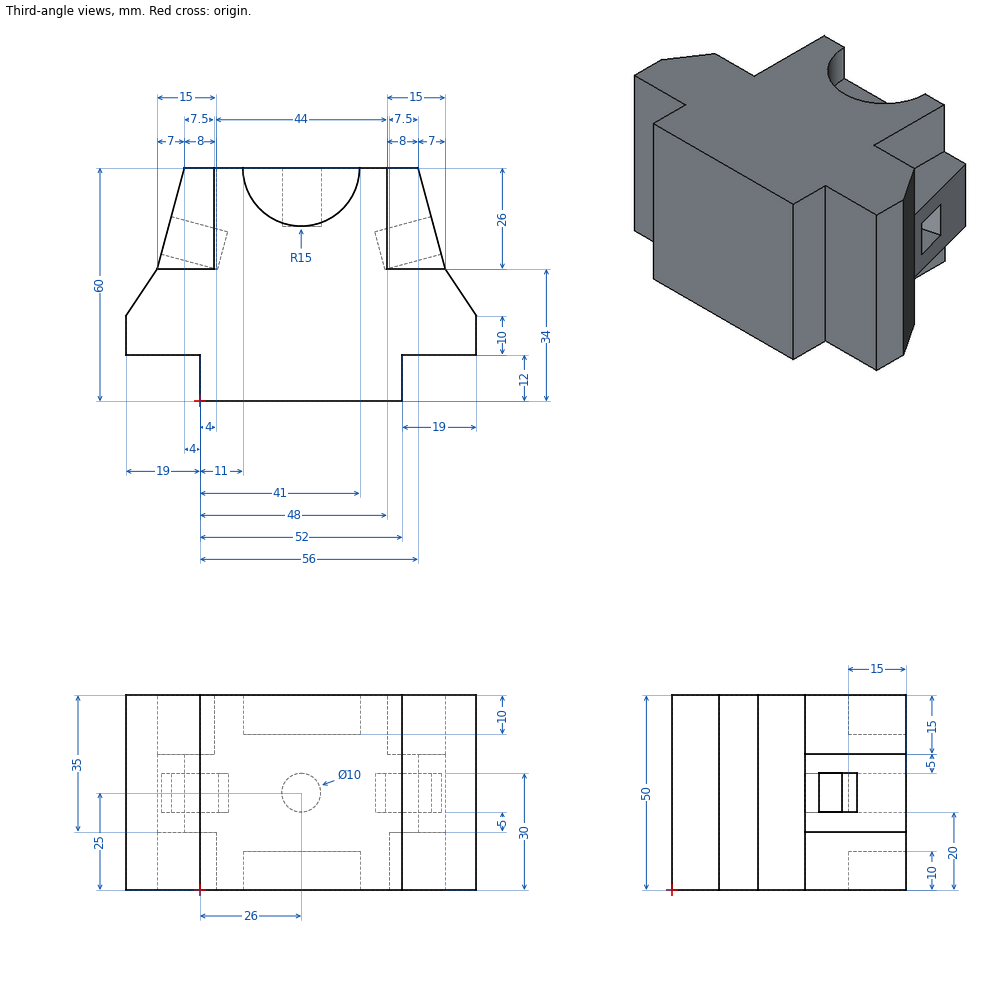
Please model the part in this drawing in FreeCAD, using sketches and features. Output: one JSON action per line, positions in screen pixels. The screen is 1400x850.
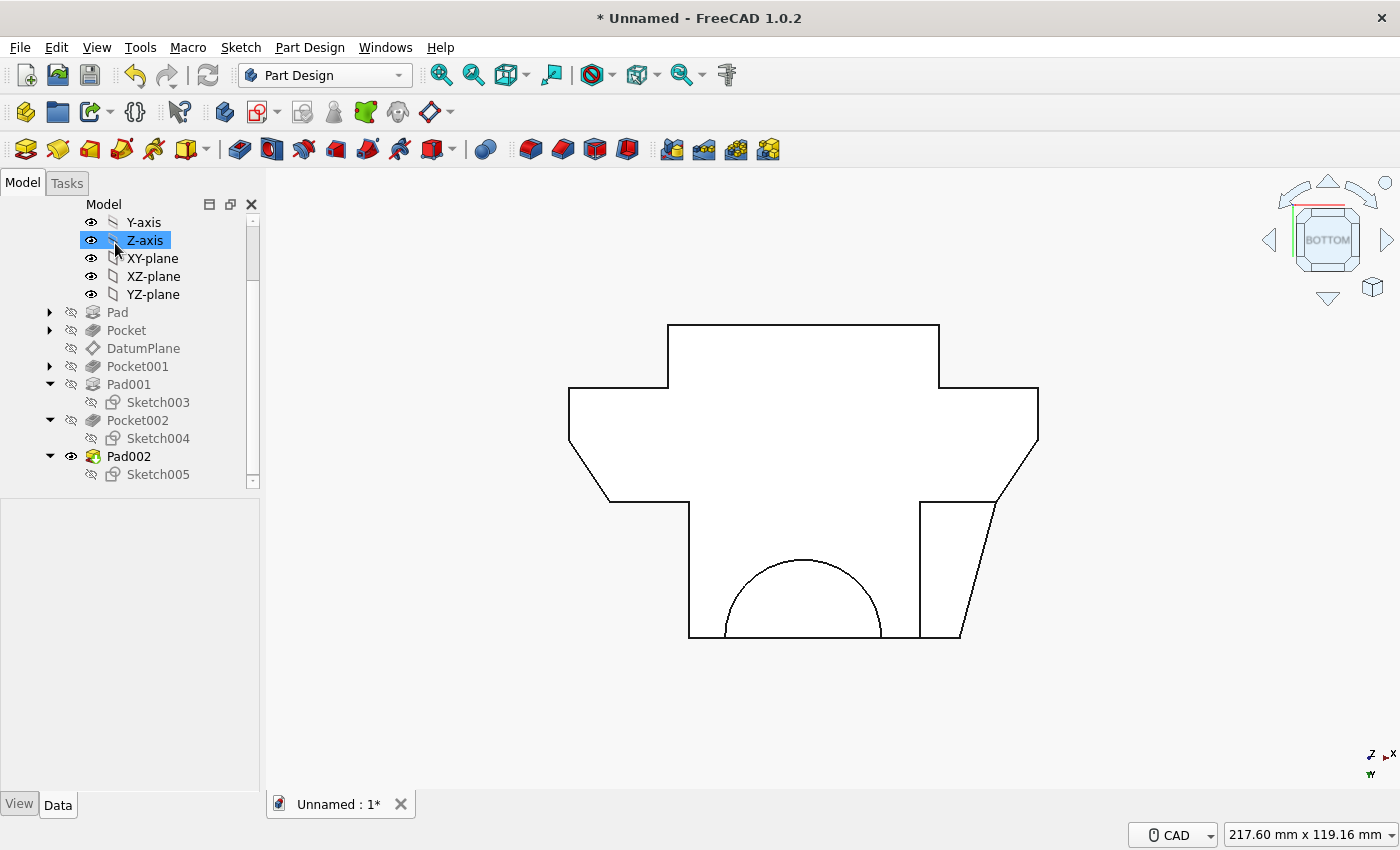
{"action": "key", "text": "0"}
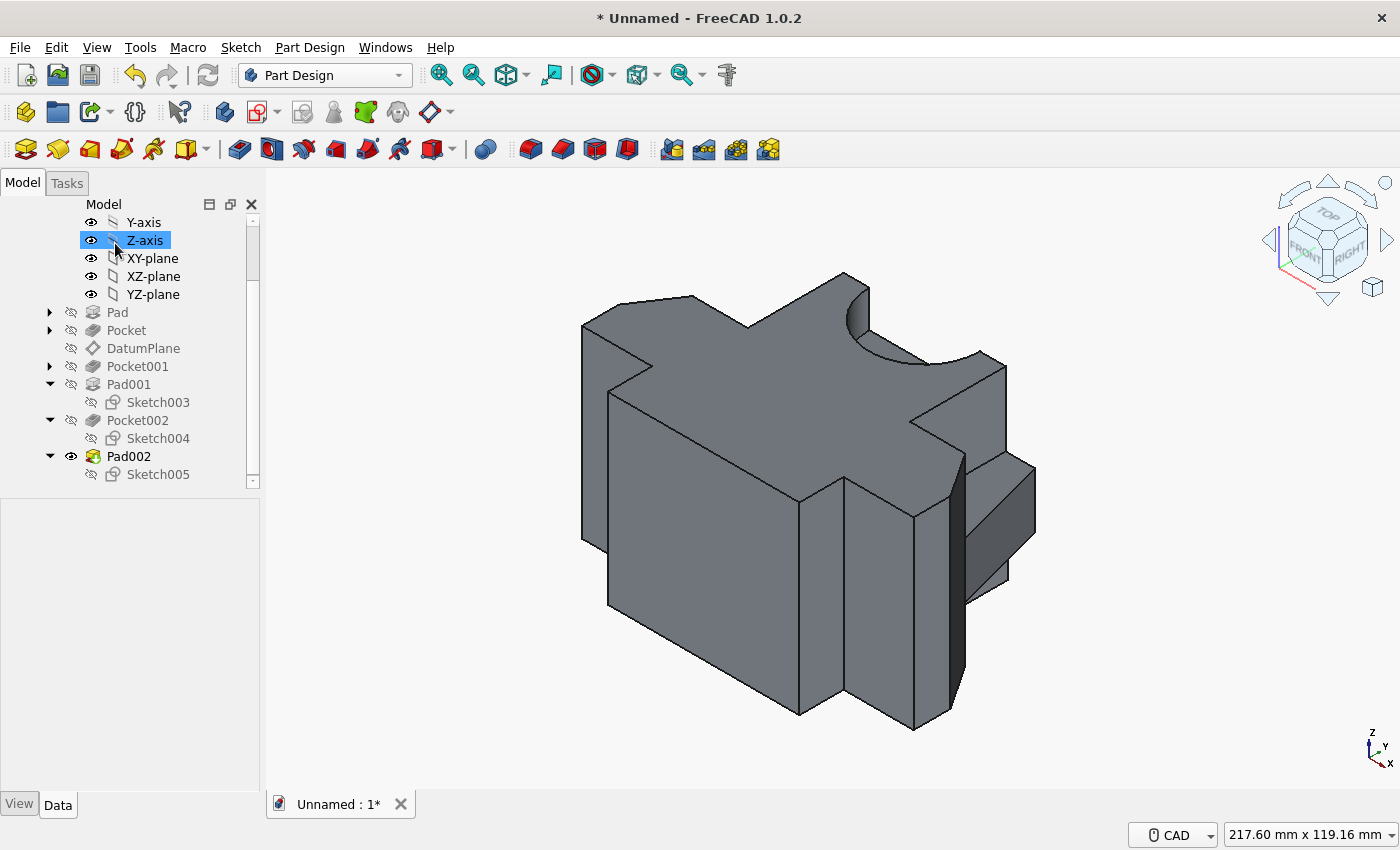
{"action": "left_click", "coordinate": [978, 490]}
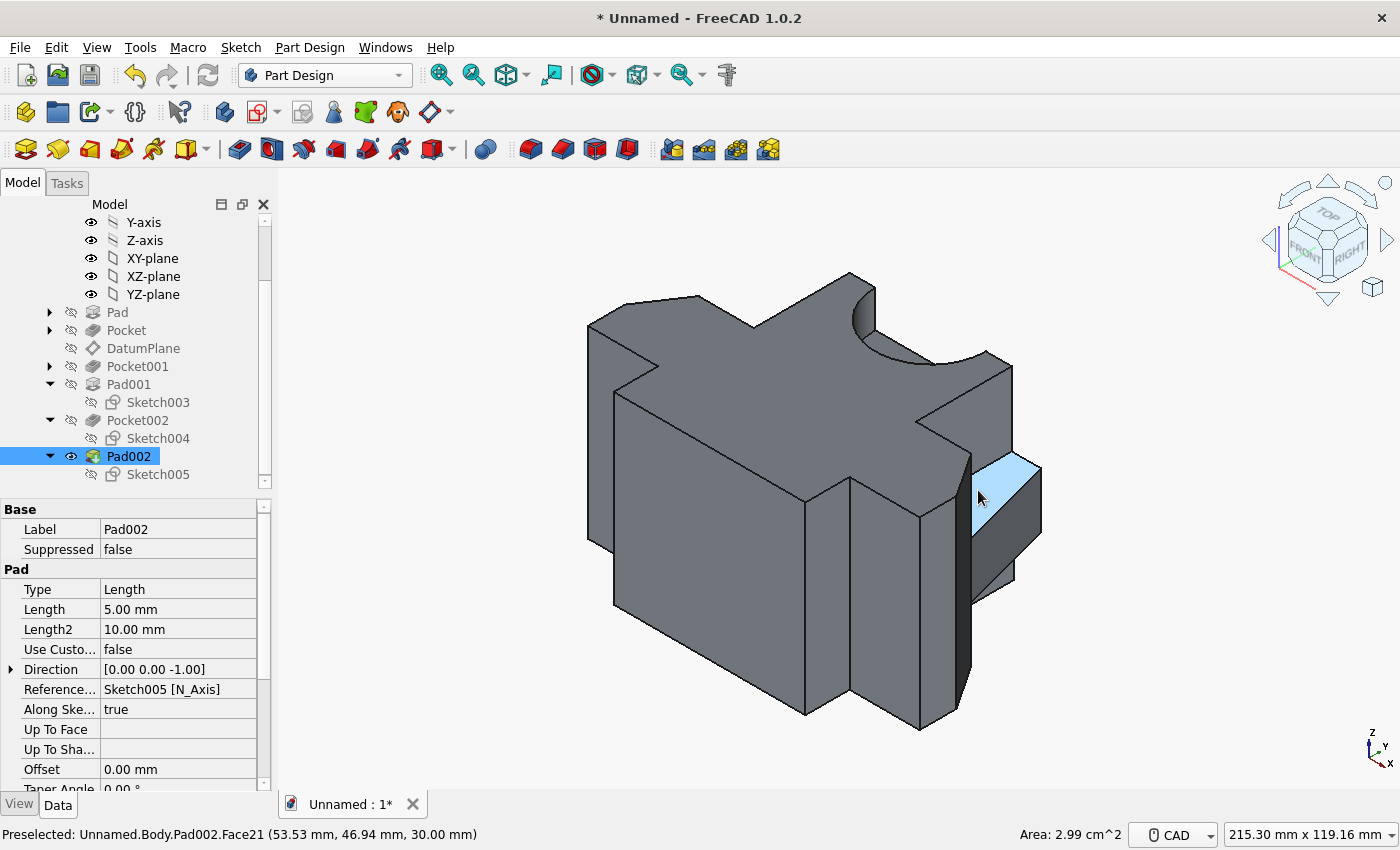
{"action": "left_click", "coordinate": [258, 112]}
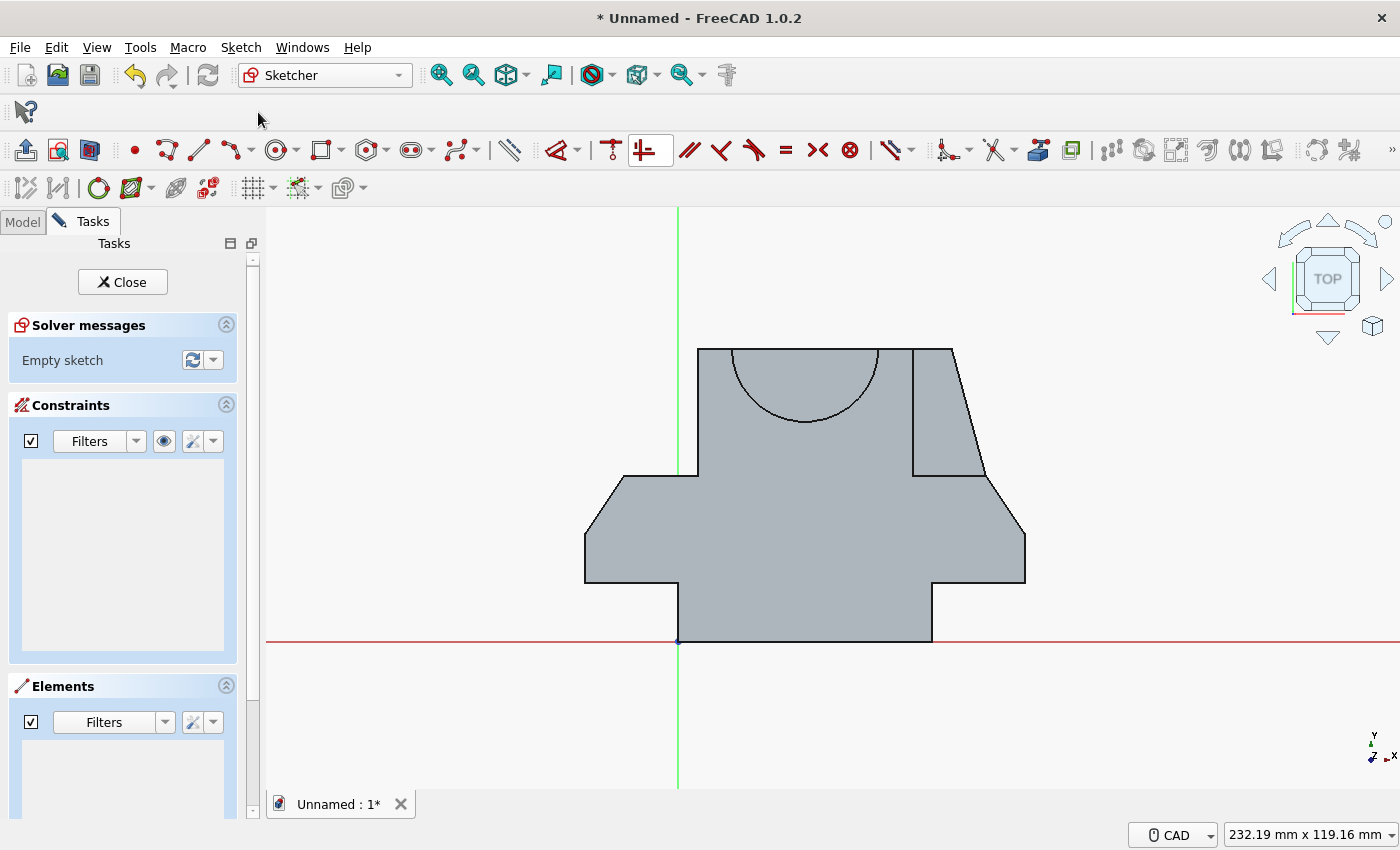
{"action": "left_click", "coordinate": [90, 150]}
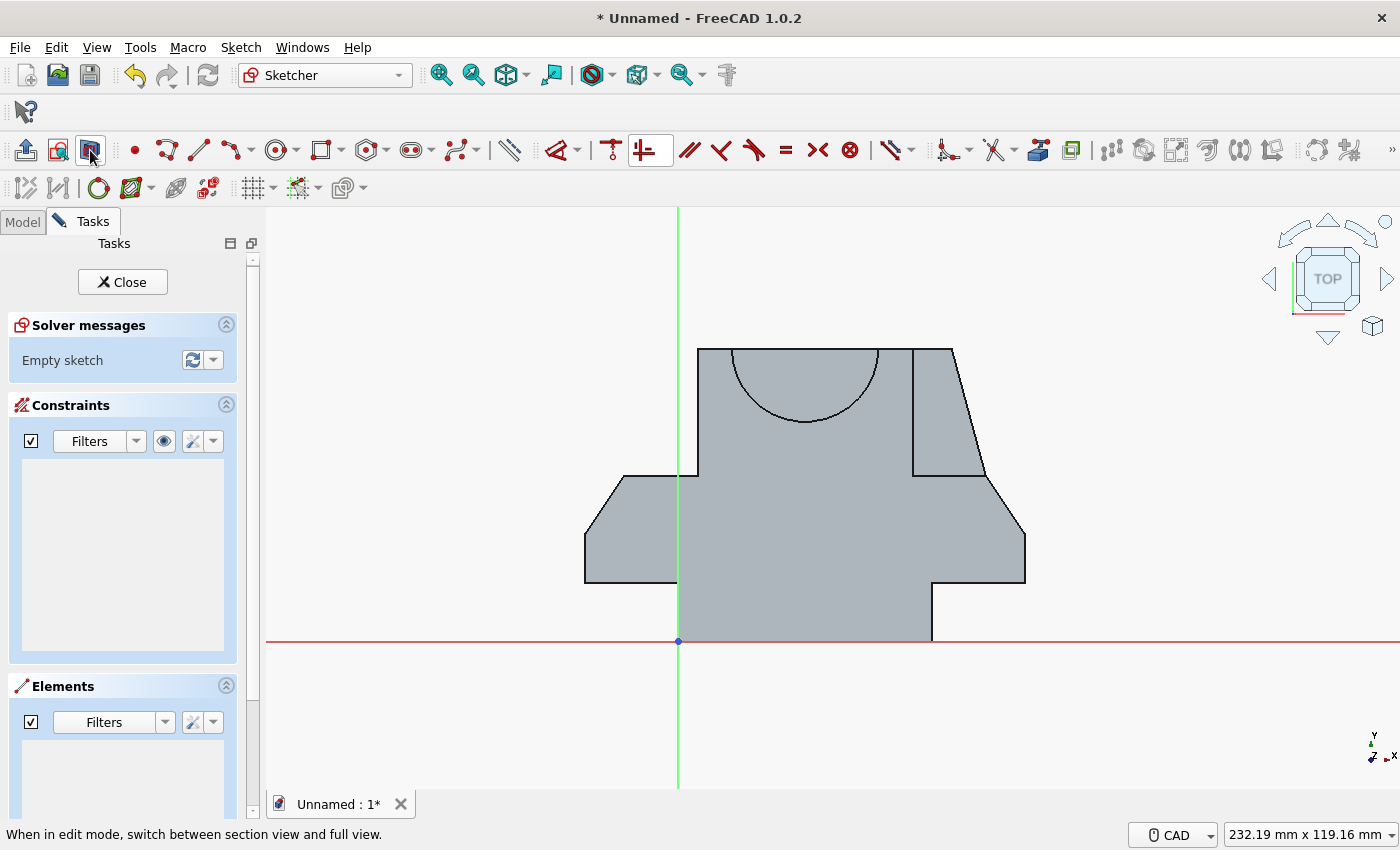
{"action": "left_click", "coordinate": [168, 150]}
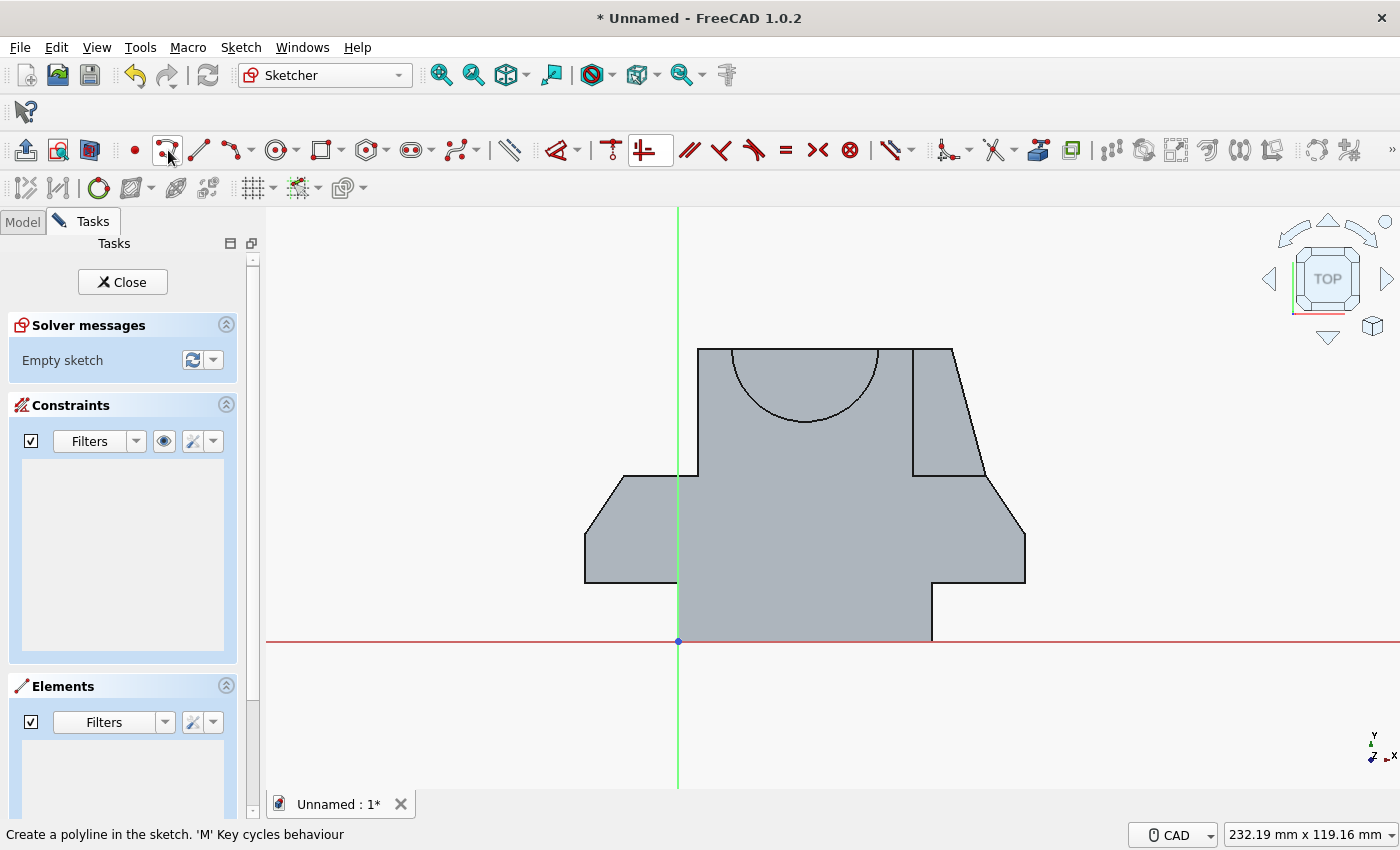
{"action": "left_click", "coordinate": [913, 476]}
{"action": "left_click", "coordinate": [986, 476]}
{"action": "left_click", "coordinate": [952, 349]}
{"action": "left_click", "coordinate": [913, 349]}
{"action": "left_click", "coordinate": [913, 477]}
{"action": "key", "text": "Escape"}
{"action": "key", "text": "Escape"}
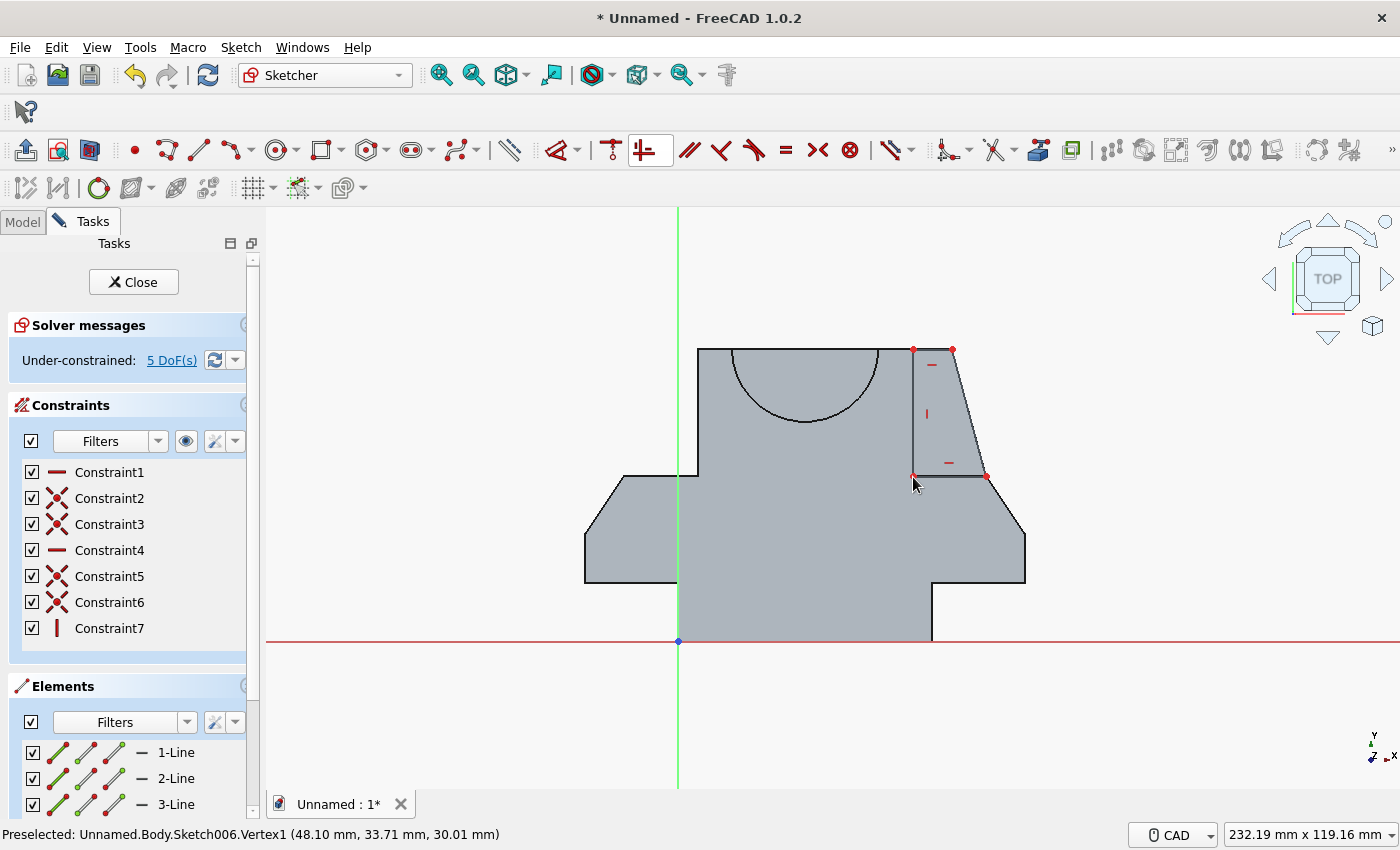
{"action": "left_click", "coordinate": [556, 150]}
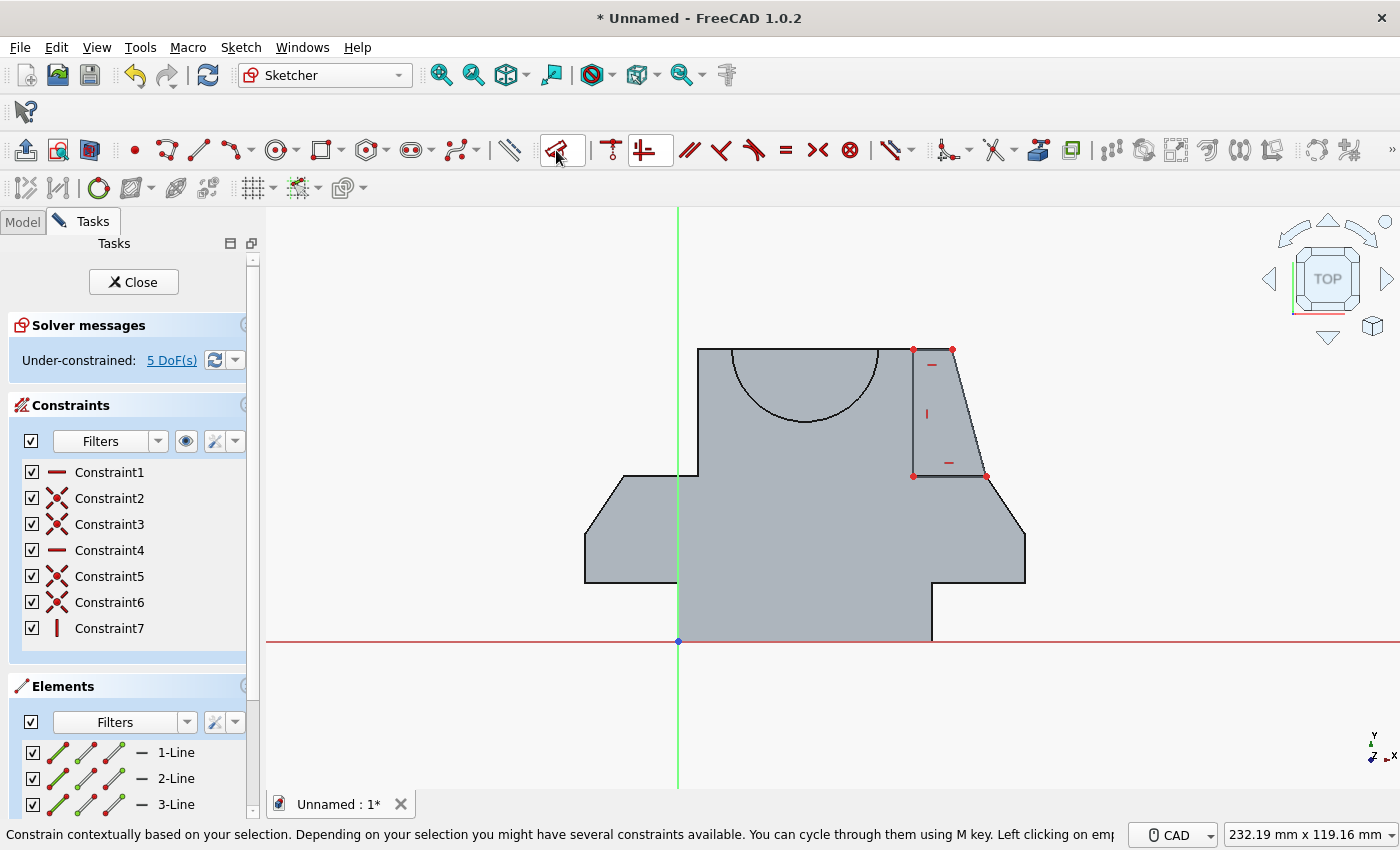
{"action": "left_click", "coordinate": [940, 350]}
{"action": "left_click", "coordinate": [933, 316]}